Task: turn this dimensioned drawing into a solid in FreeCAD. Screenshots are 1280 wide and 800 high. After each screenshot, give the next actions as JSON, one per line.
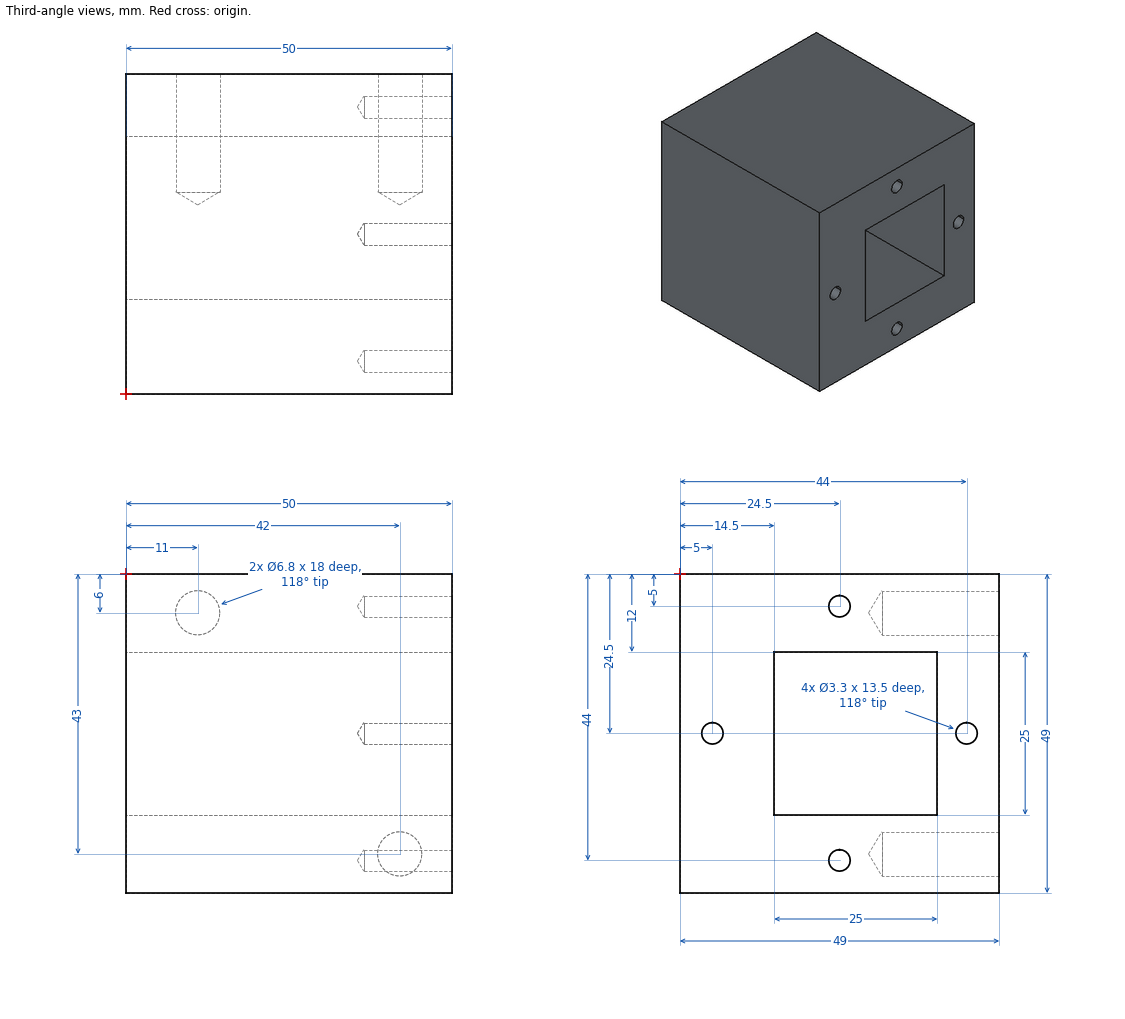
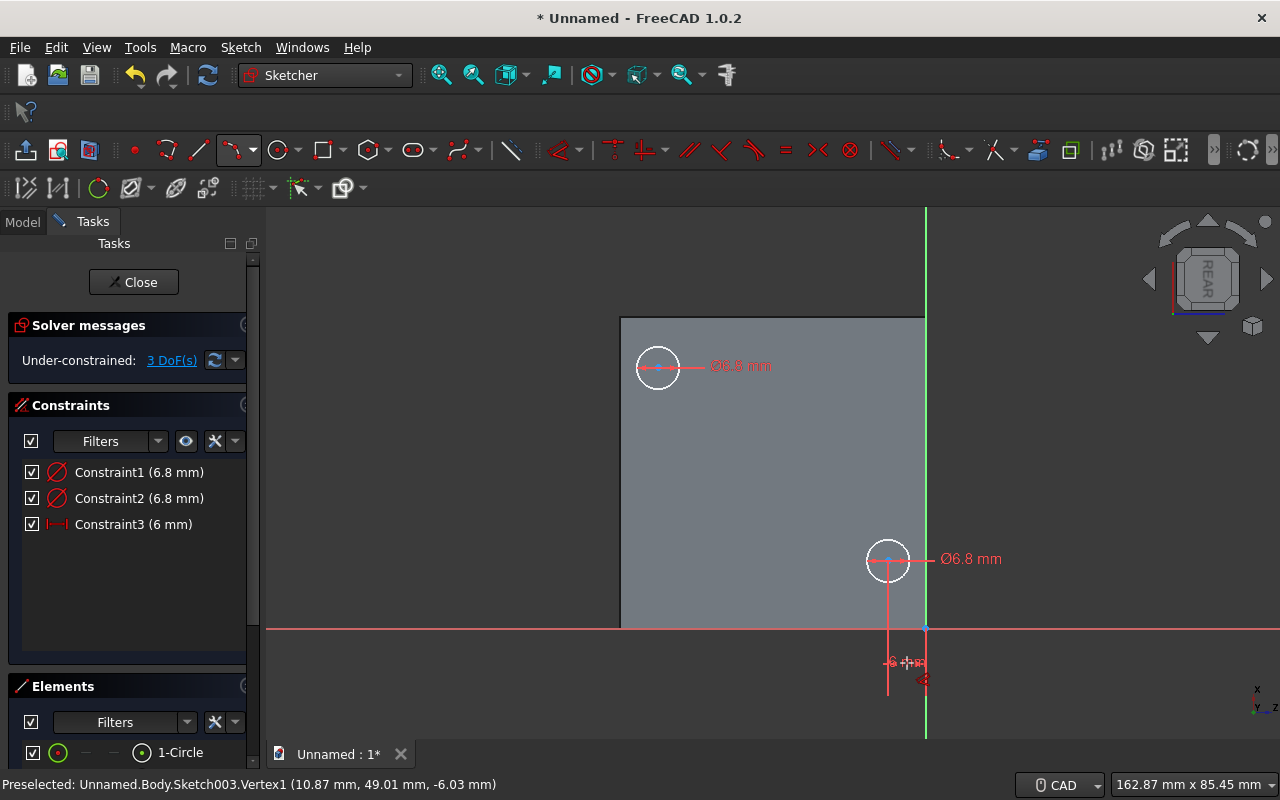
{"action": "left_click", "coordinate": [888, 561]}
{"action": "left_click", "coordinate": [960, 595]}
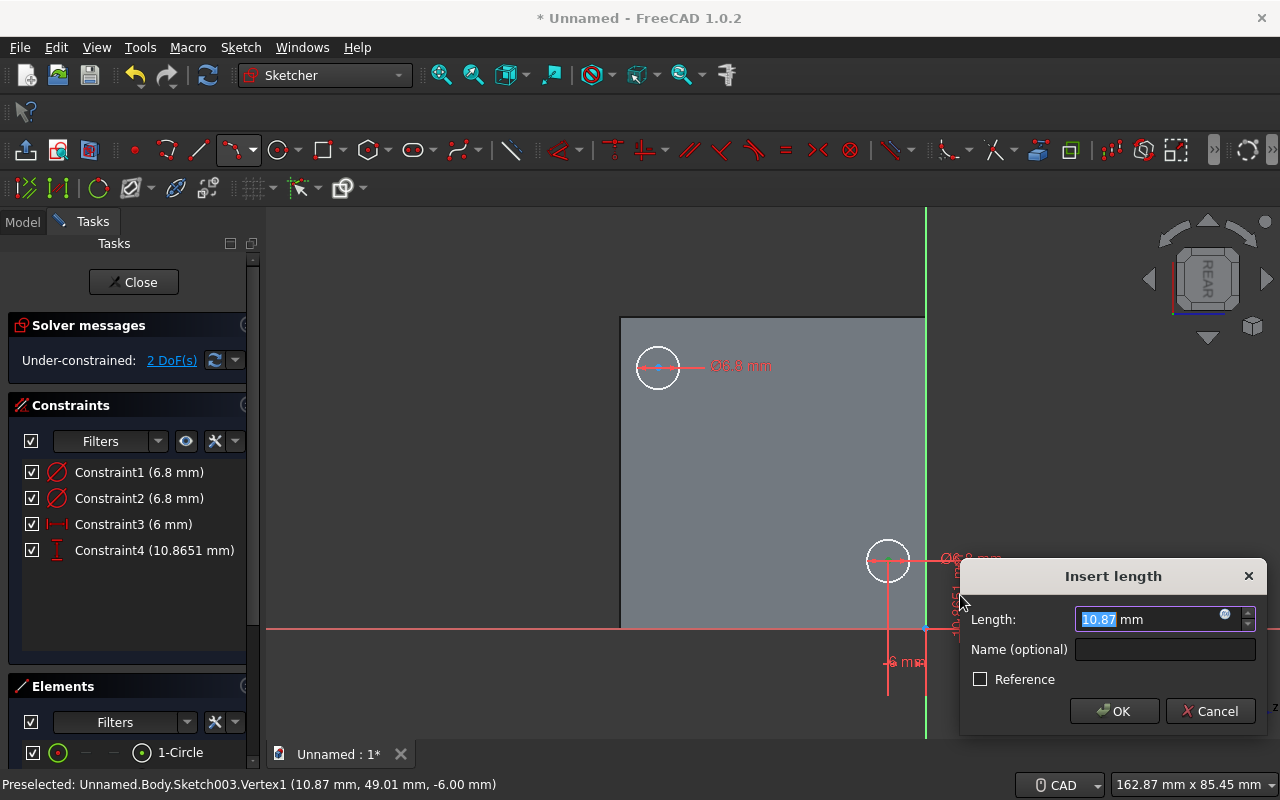
{"action": "type", "text": "11"}
{"action": "key", "text": "Return"}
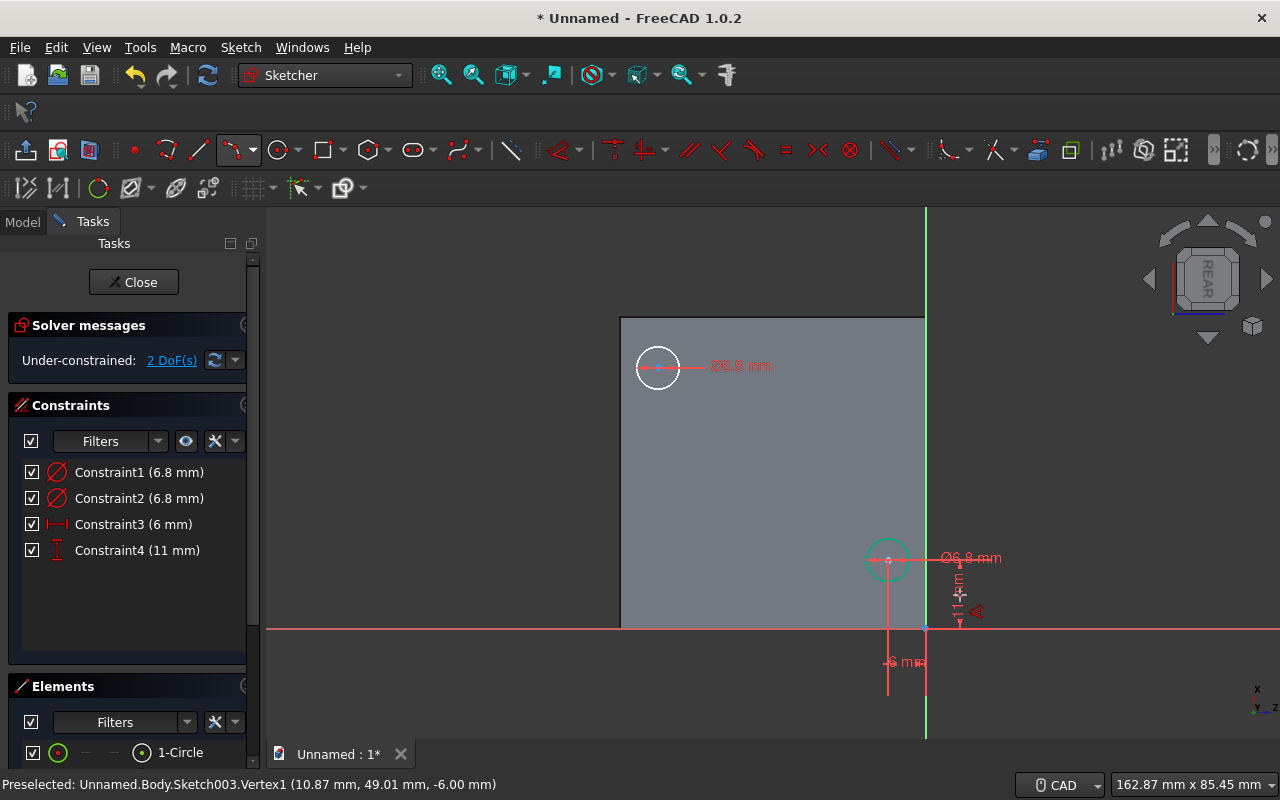
{"action": "left_click", "coordinate": [658, 368]}
{"action": "left_click", "coordinate": [792, 663]}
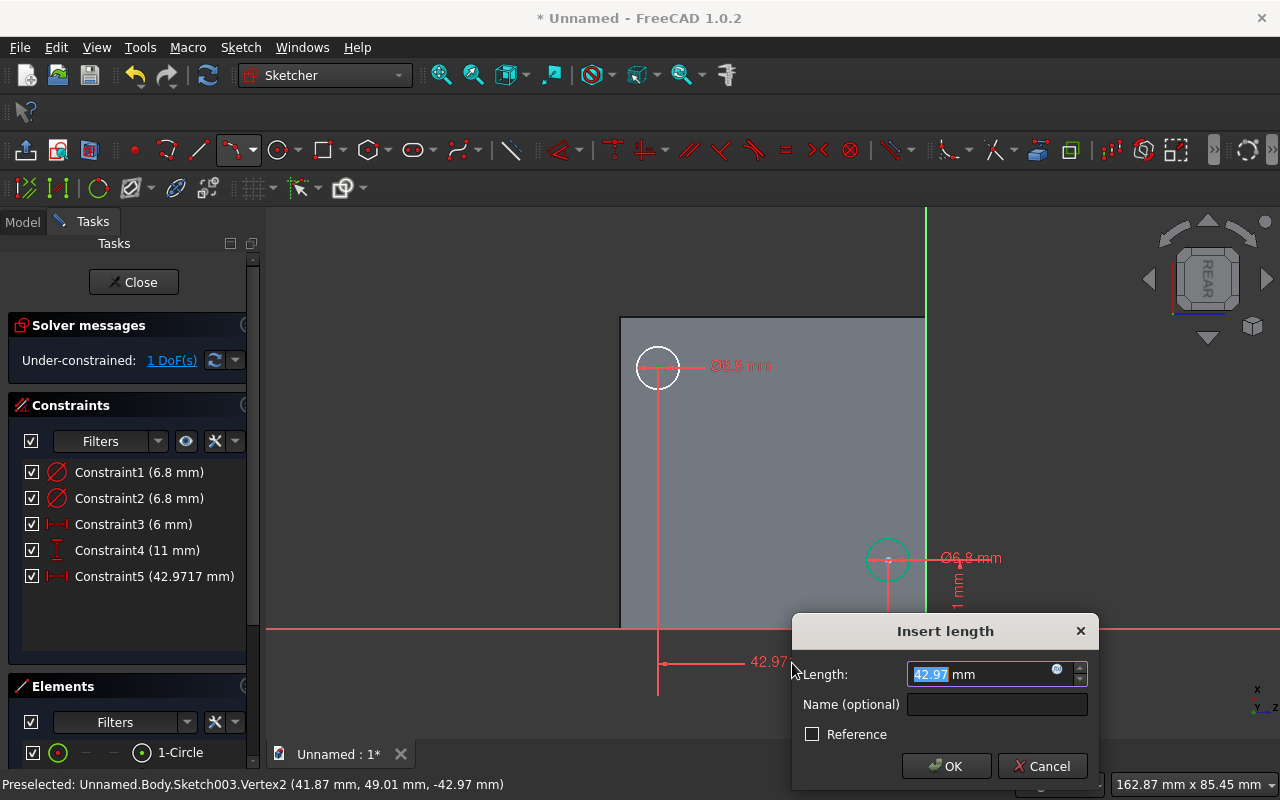
{"action": "type", "text": "43"}
{"action": "key", "text": "Return"}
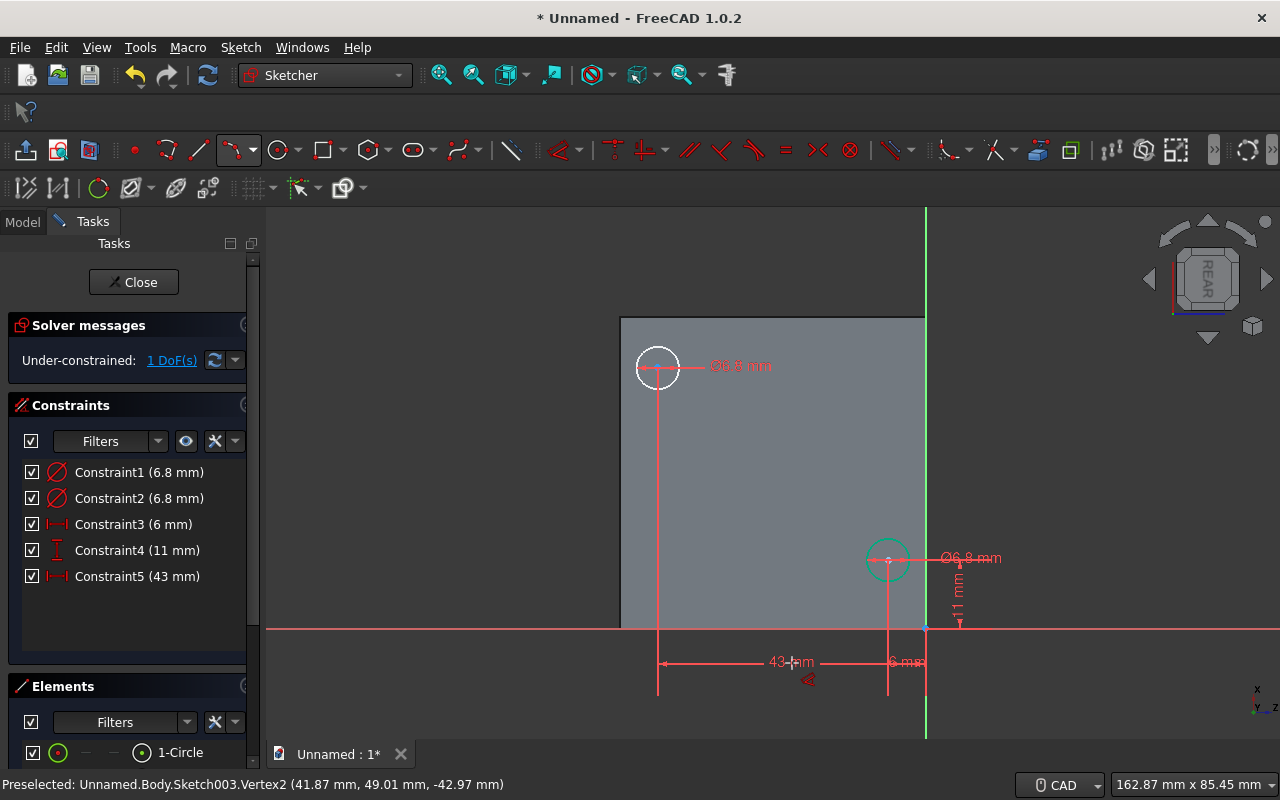
{"action": "left_click", "coordinate": [658, 368]}
{"action": "left_click", "coordinate": [960, 498]}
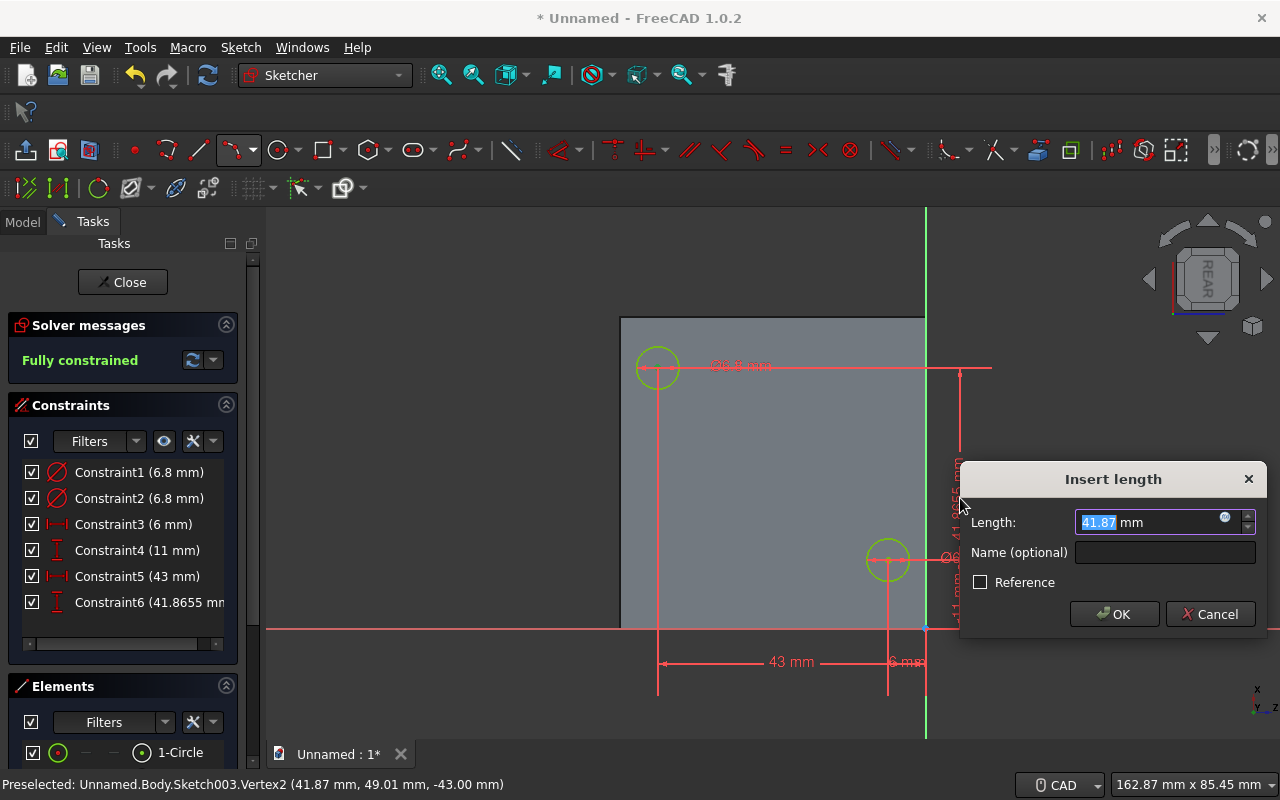
{"action": "type", "text": "42"}
{"action": "key", "text": "Return"}
{"action": "key", "text": "Escape"}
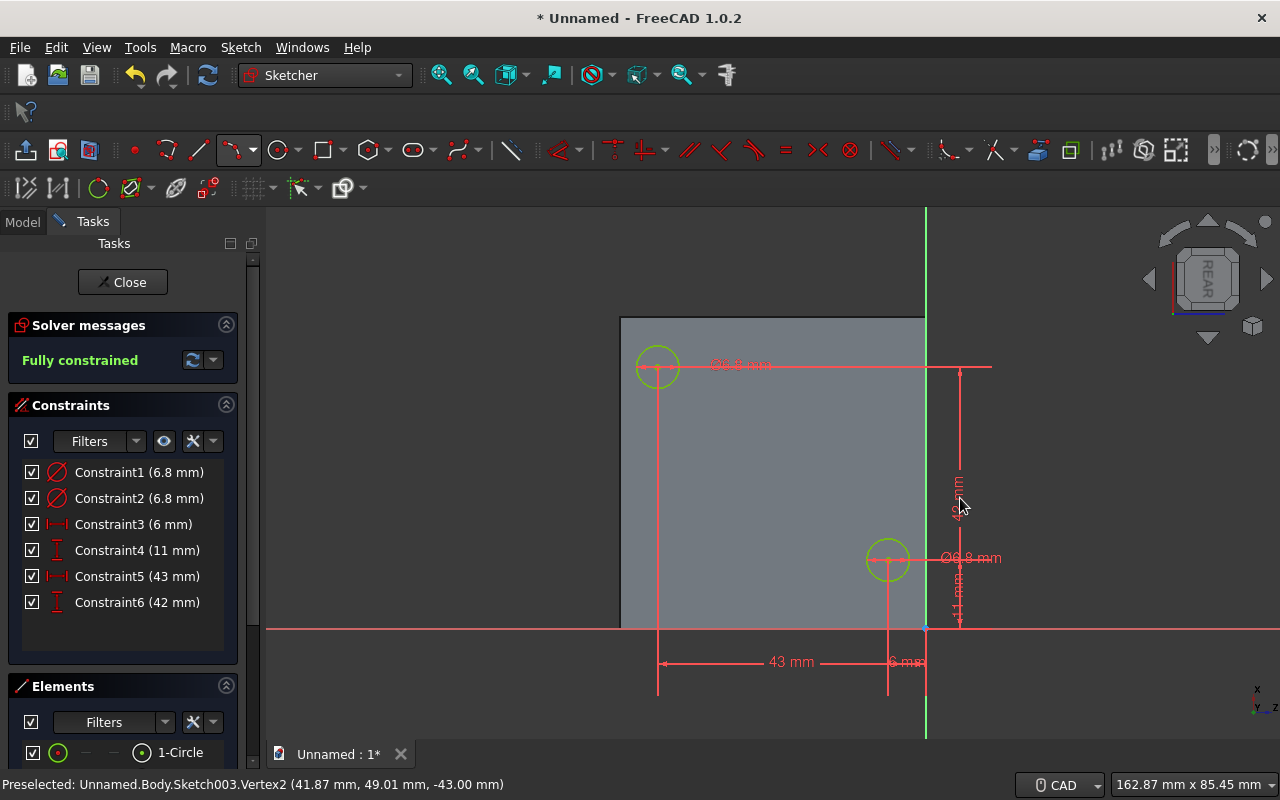
{"action": "left_click", "coordinate": [123, 282]}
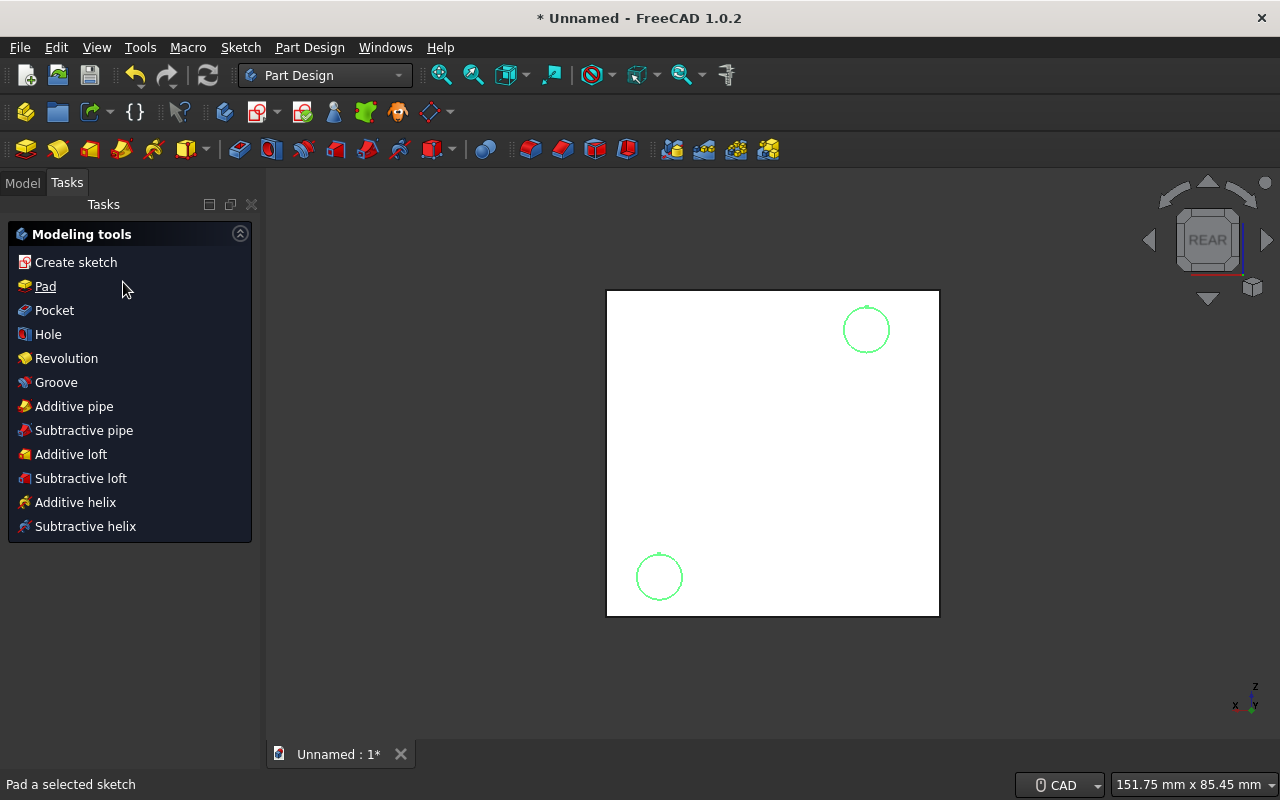
{"action": "left_click", "coordinate": [272, 150]}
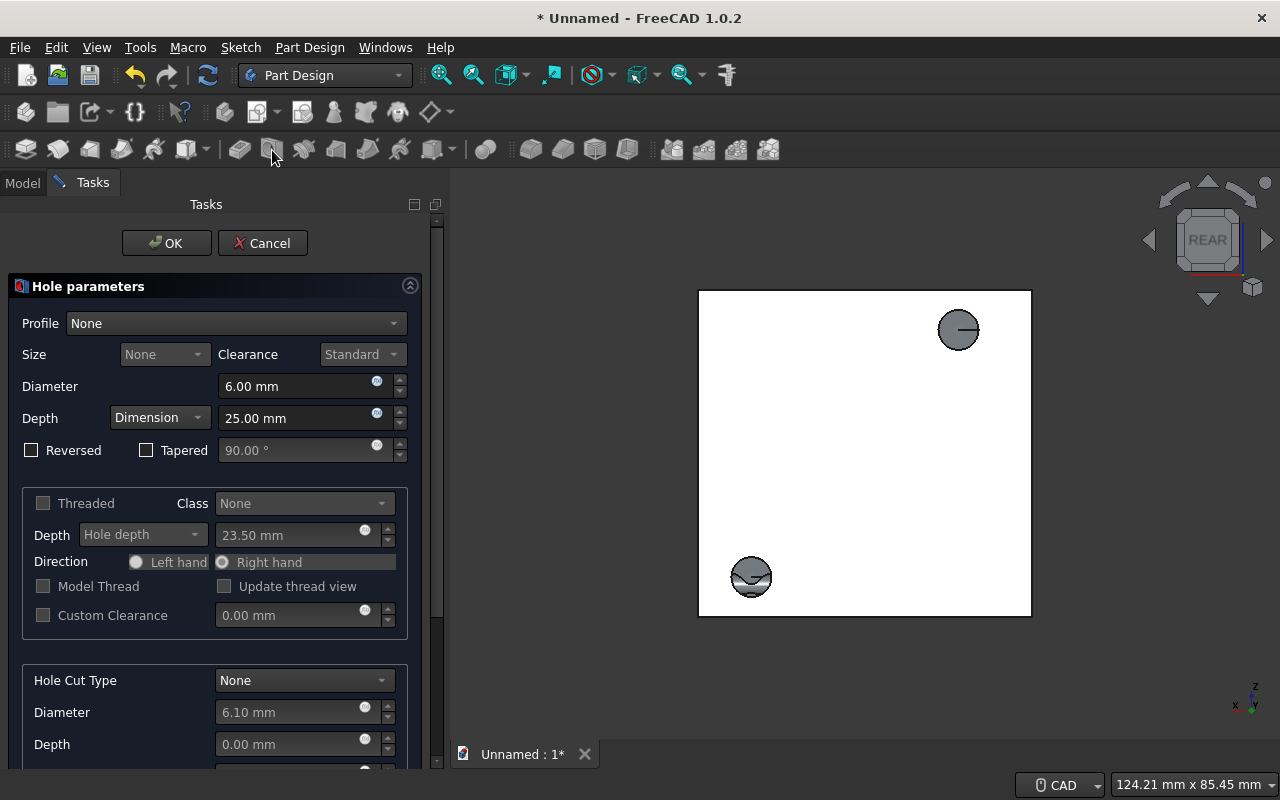
{"action": "triple_click", "coordinate": [305, 386]}